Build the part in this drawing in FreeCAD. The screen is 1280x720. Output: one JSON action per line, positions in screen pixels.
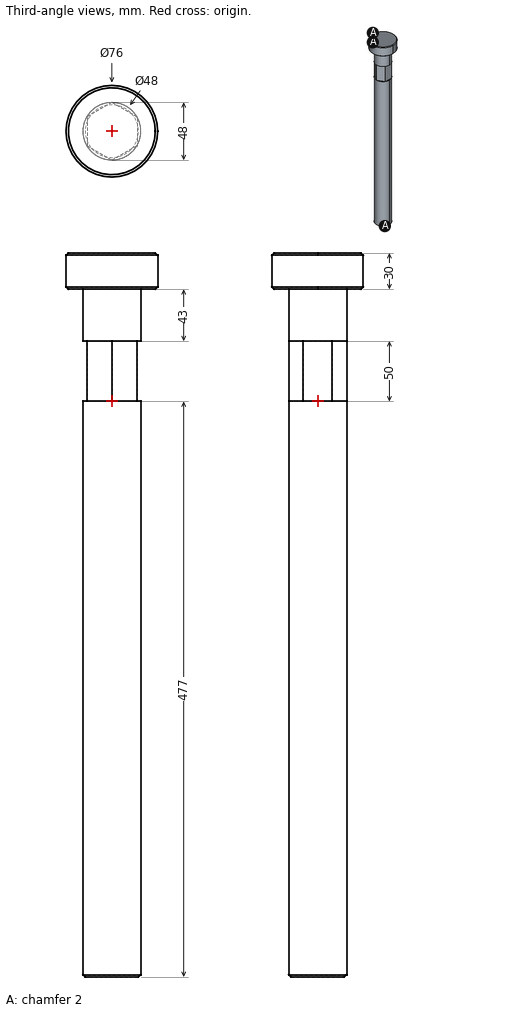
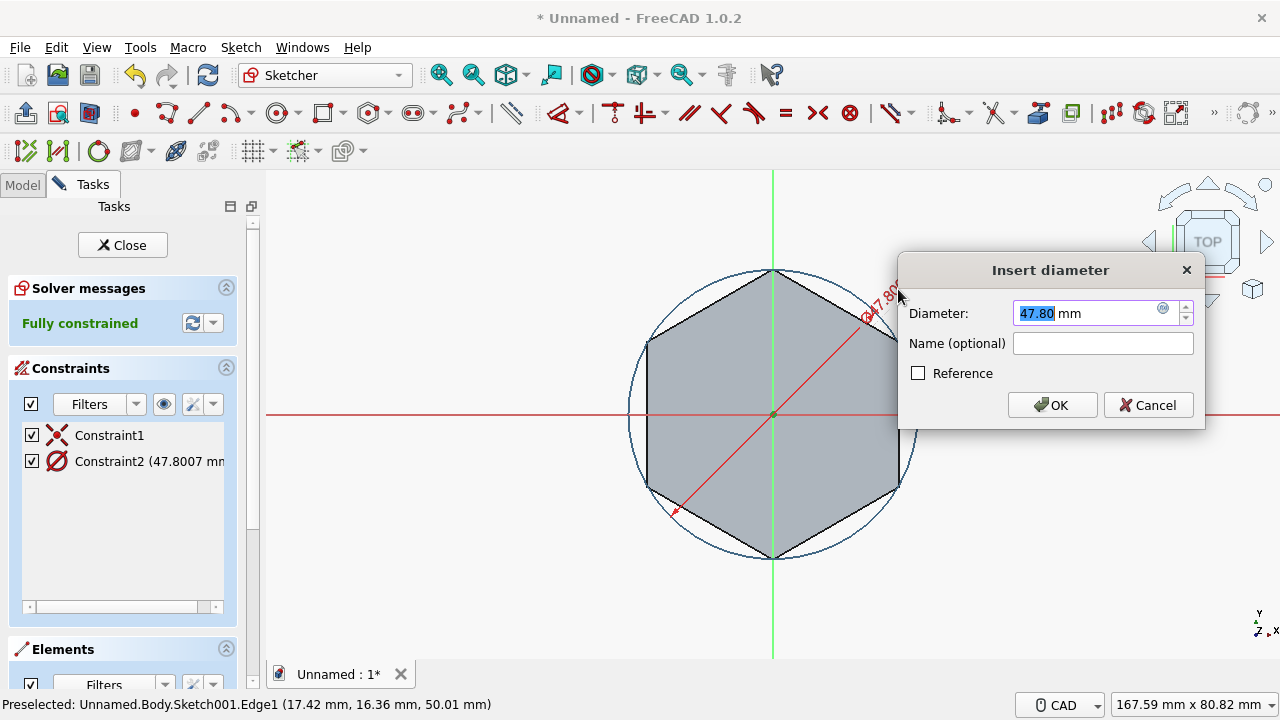
{"action": "type", "text": "48"}
{"action": "key", "text": "Return"}
{"action": "key", "text": "Escape"}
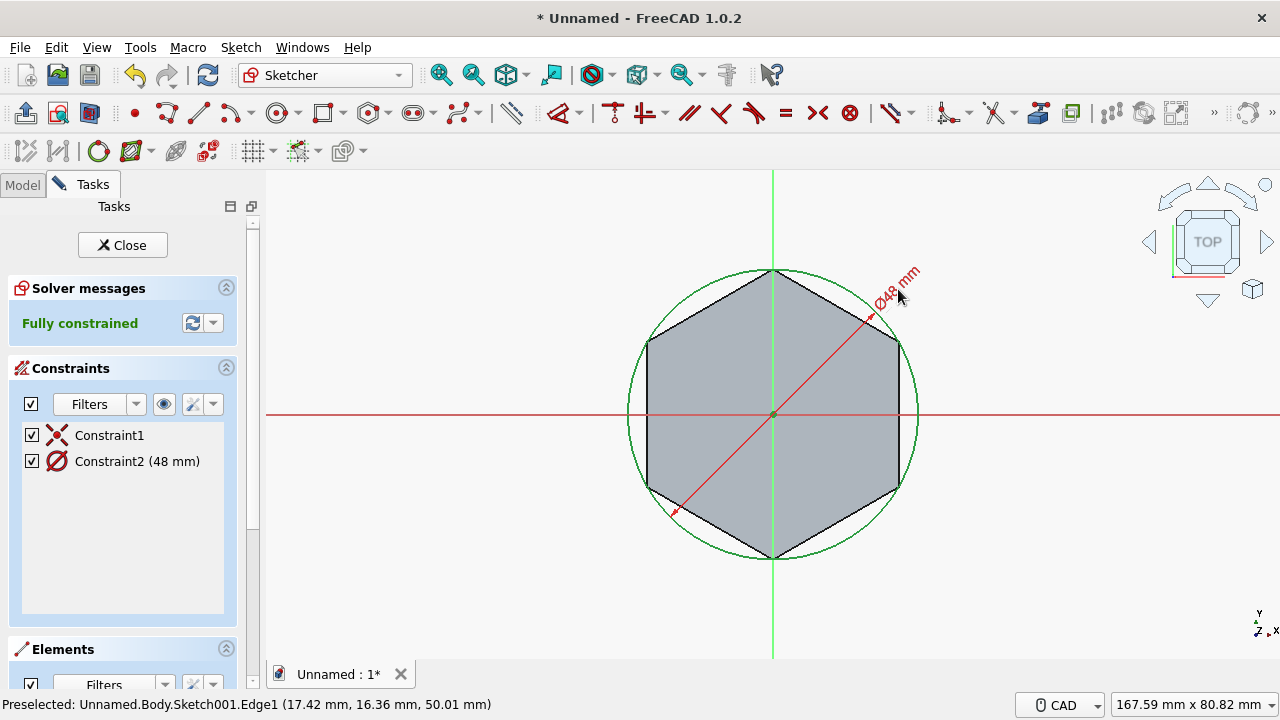
{"action": "left_click", "coordinate": [123, 245]}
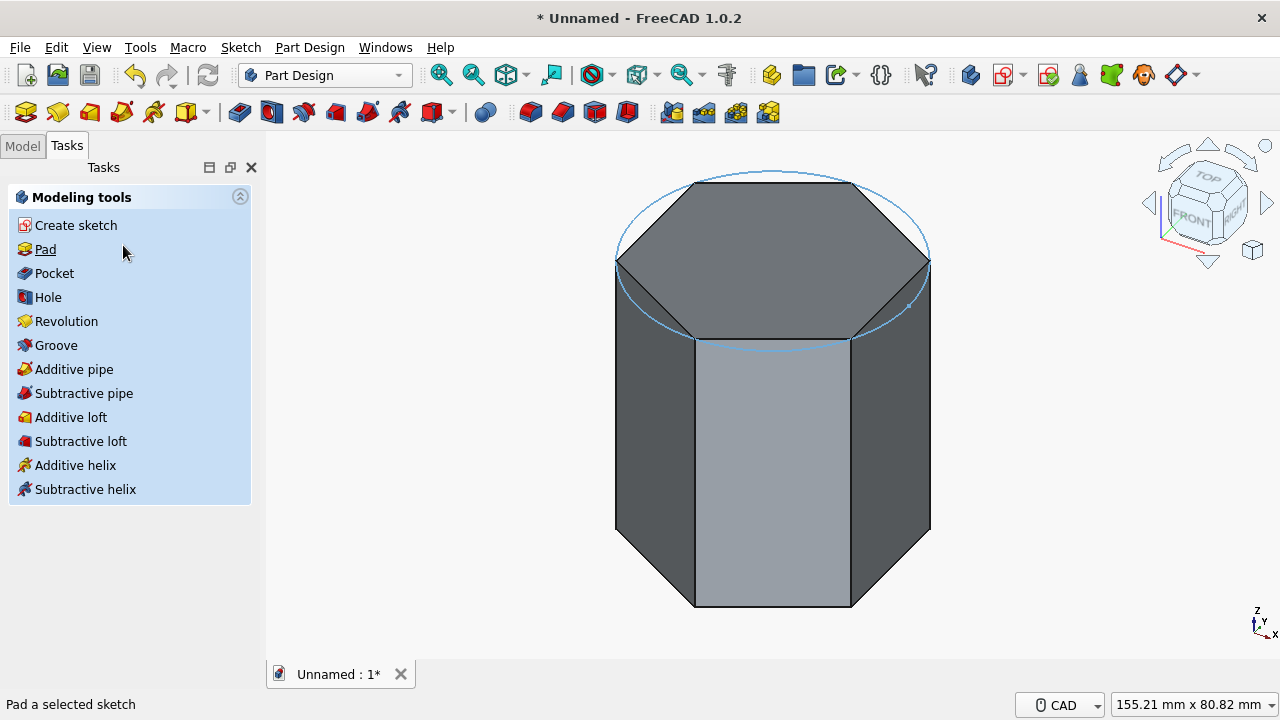
{"action": "left_click", "coordinate": [26, 112]}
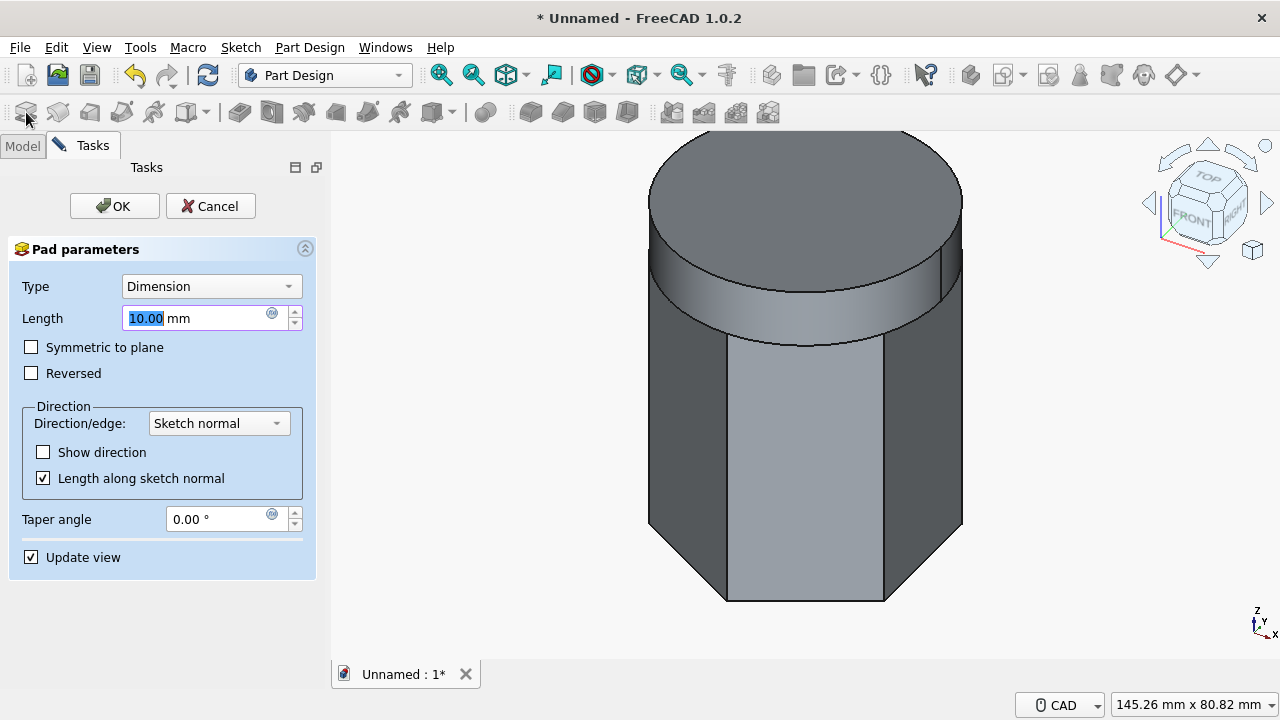
{"action": "type", "text": "43"}
{"action": "key", "text": "Tab"}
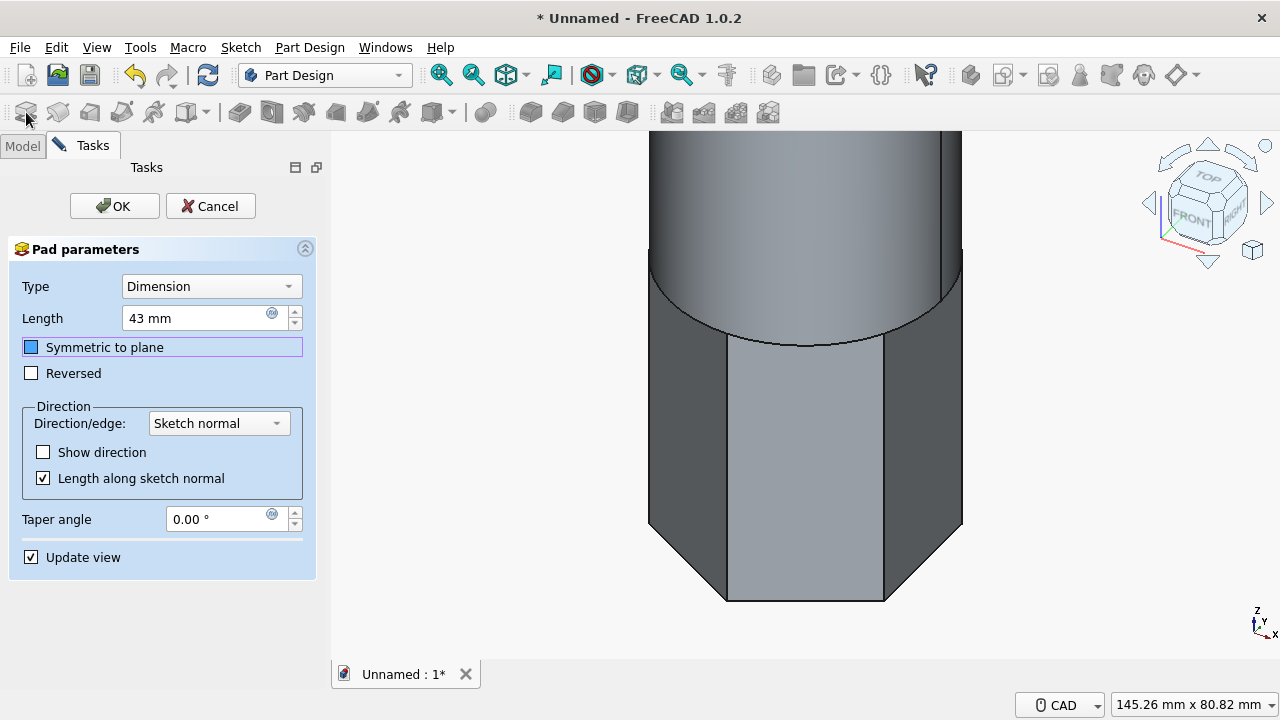
{"action": "left_click", "coordinate": [115, 206]}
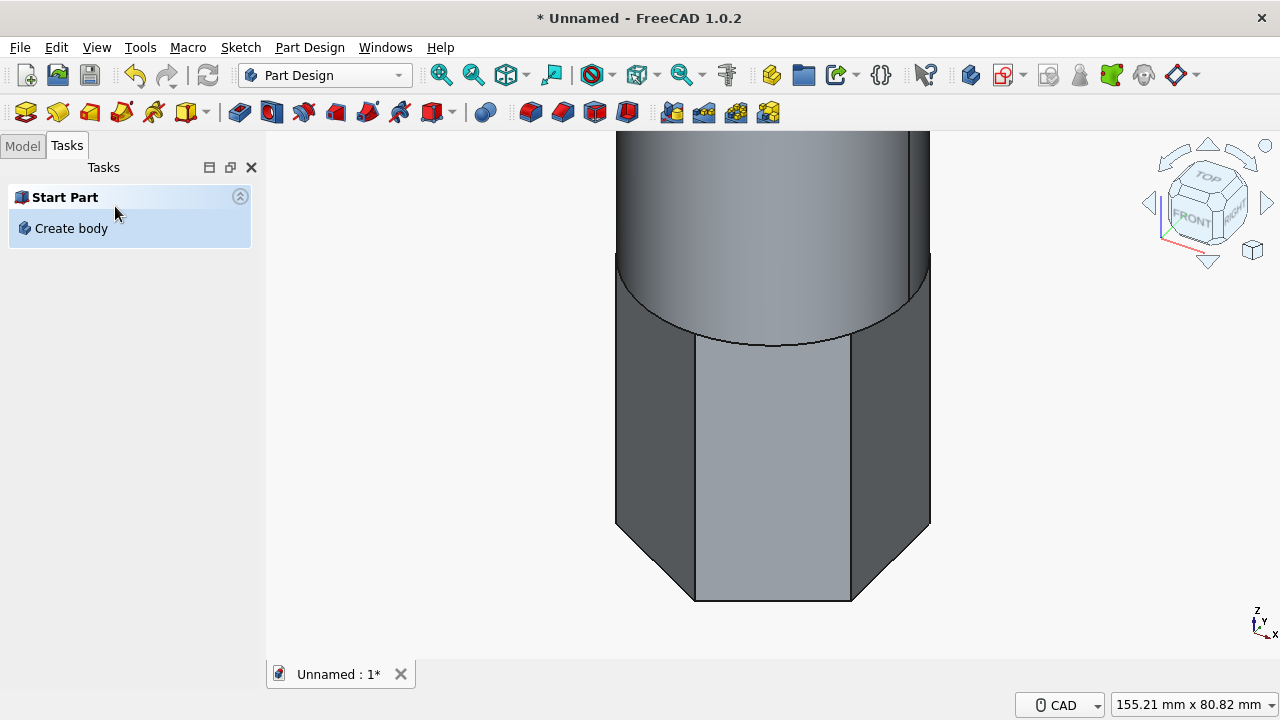
{"action": "left_click", "coordinate": [442, 76]}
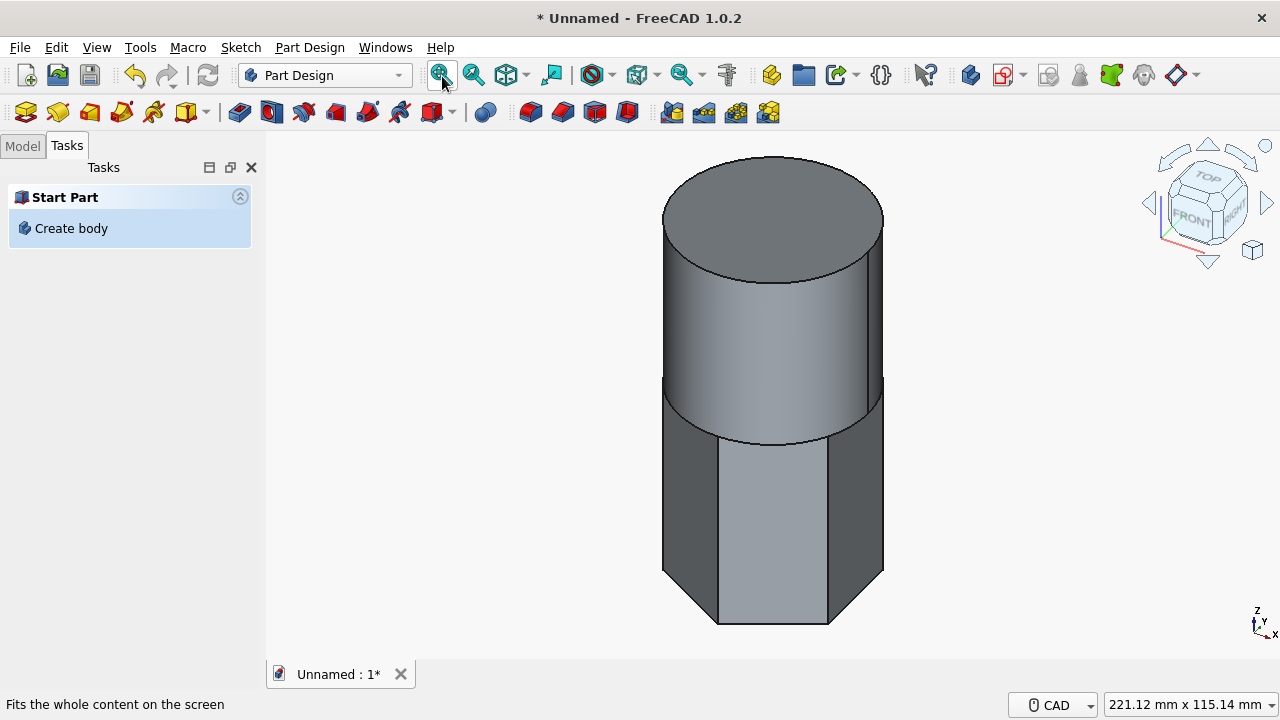
{"action": "left_click", "coordinate": [773, 219]}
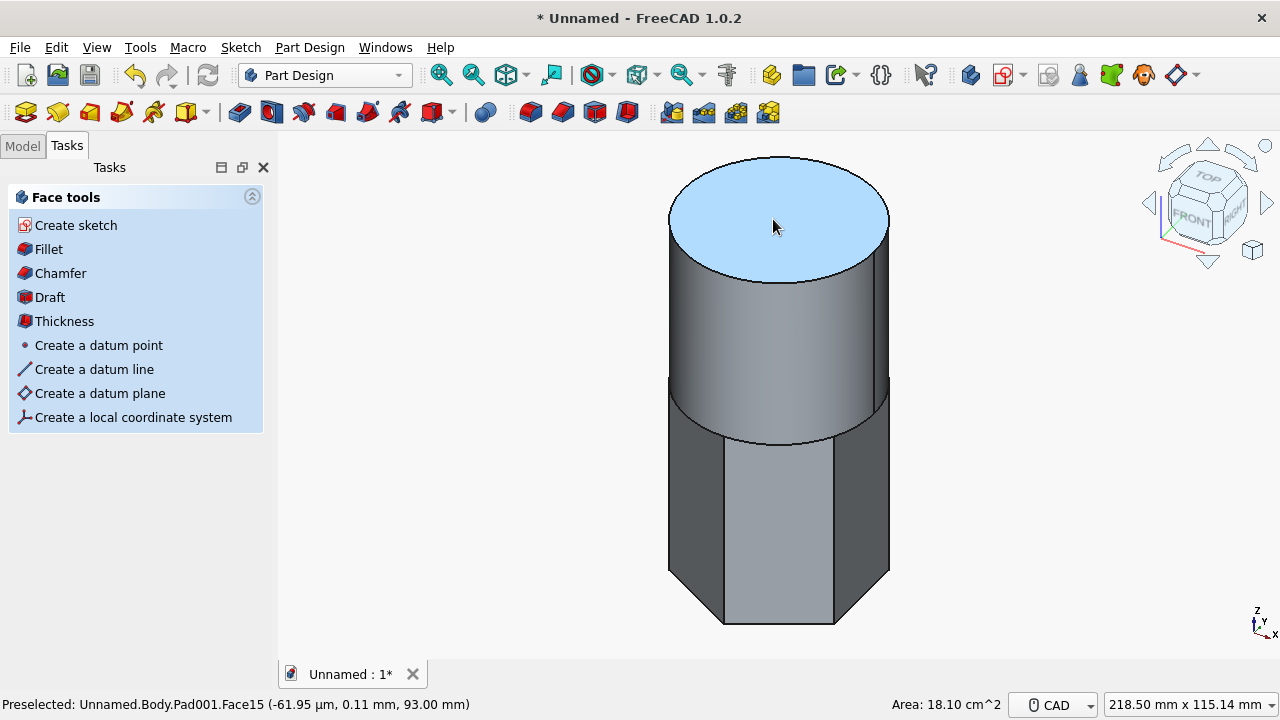
{"action": "left_click", "coordinate": [1004, 76]}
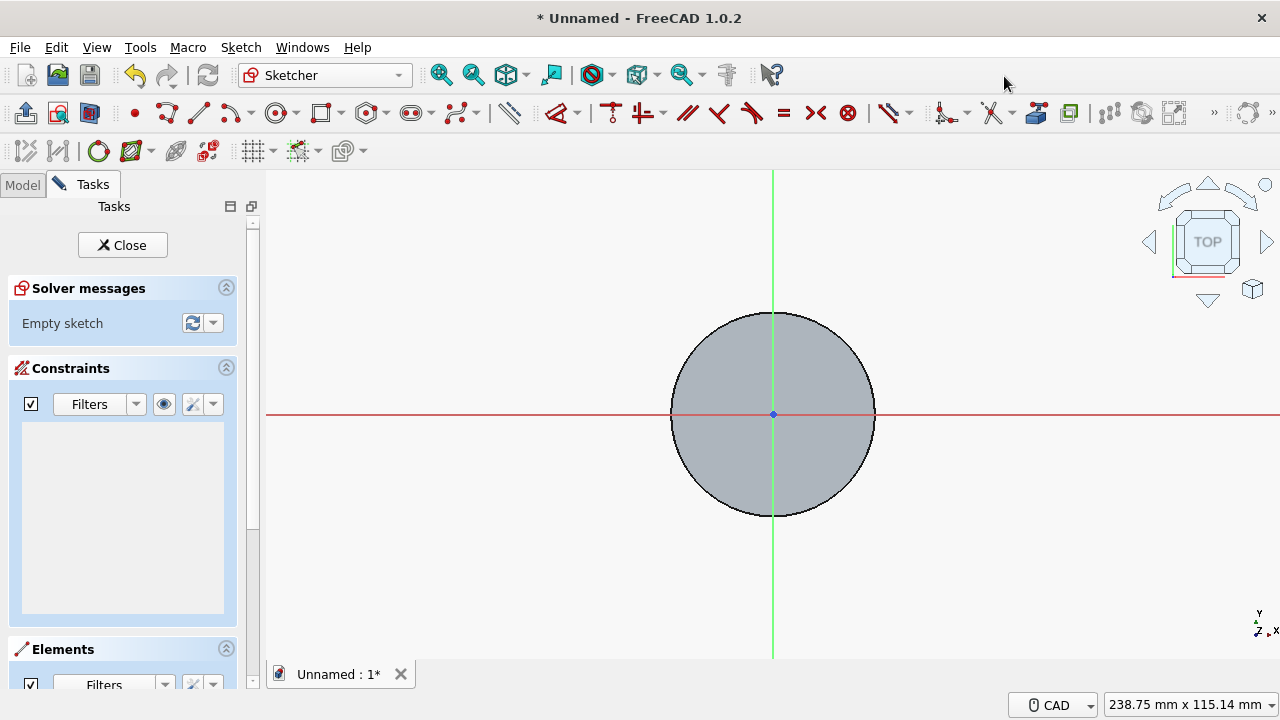
{"action": "left_click", "coordinate": [276, 114]}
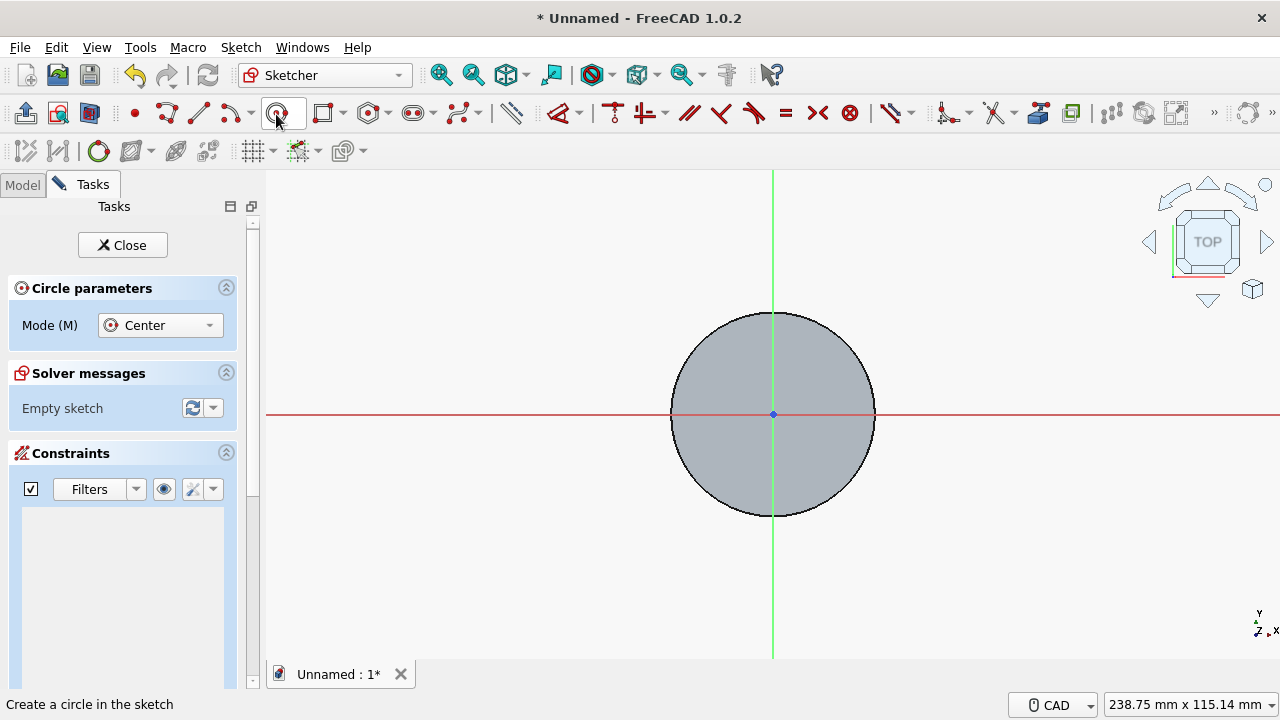
{"action": "left_click", "coordinate": [773, 414]}
{"action": "left_click", "coordinate": [887, 300]}
{"action": "key", "text": "Escape"}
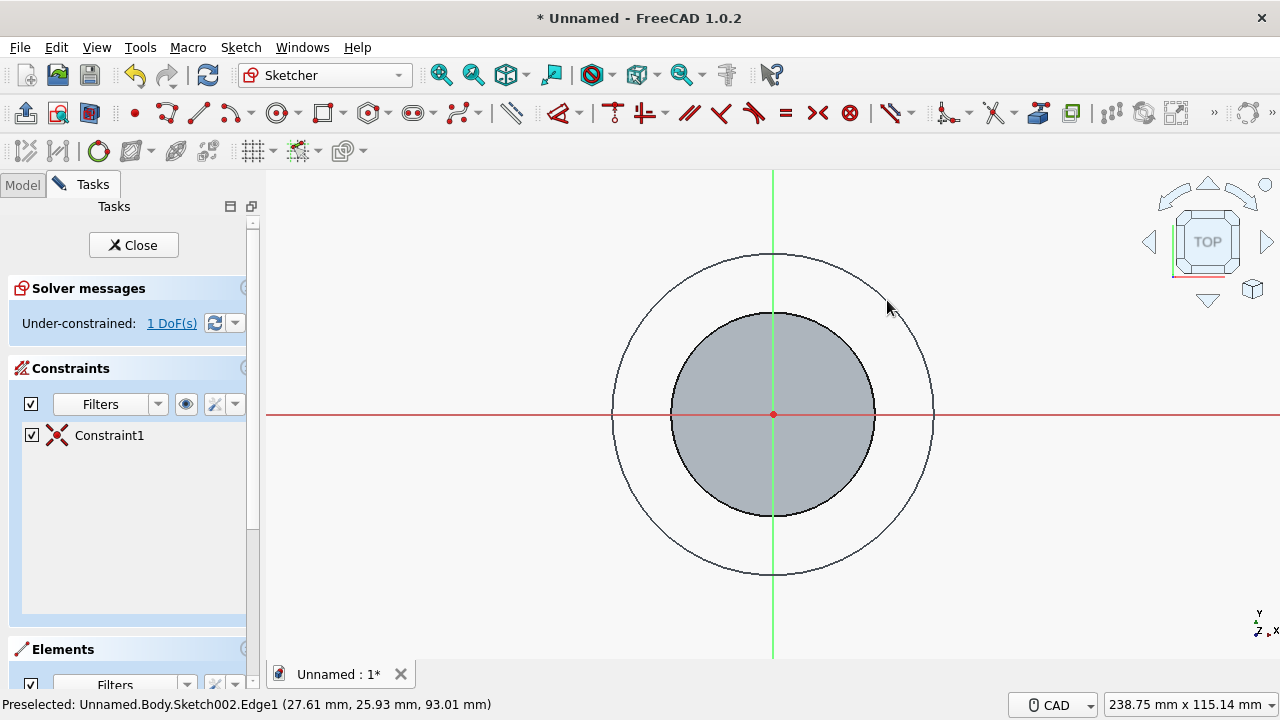
{"action": "left_click", "coordinate": [558, 114]}